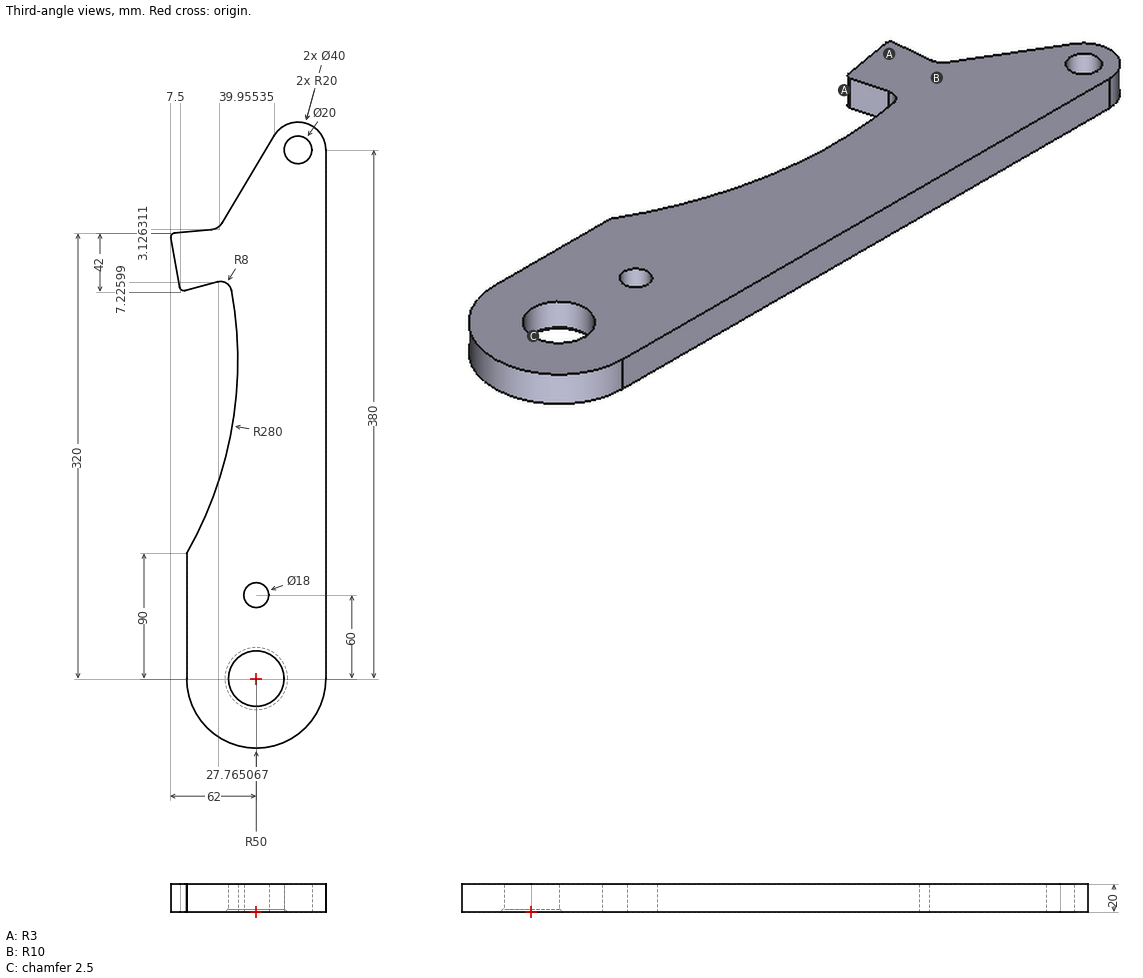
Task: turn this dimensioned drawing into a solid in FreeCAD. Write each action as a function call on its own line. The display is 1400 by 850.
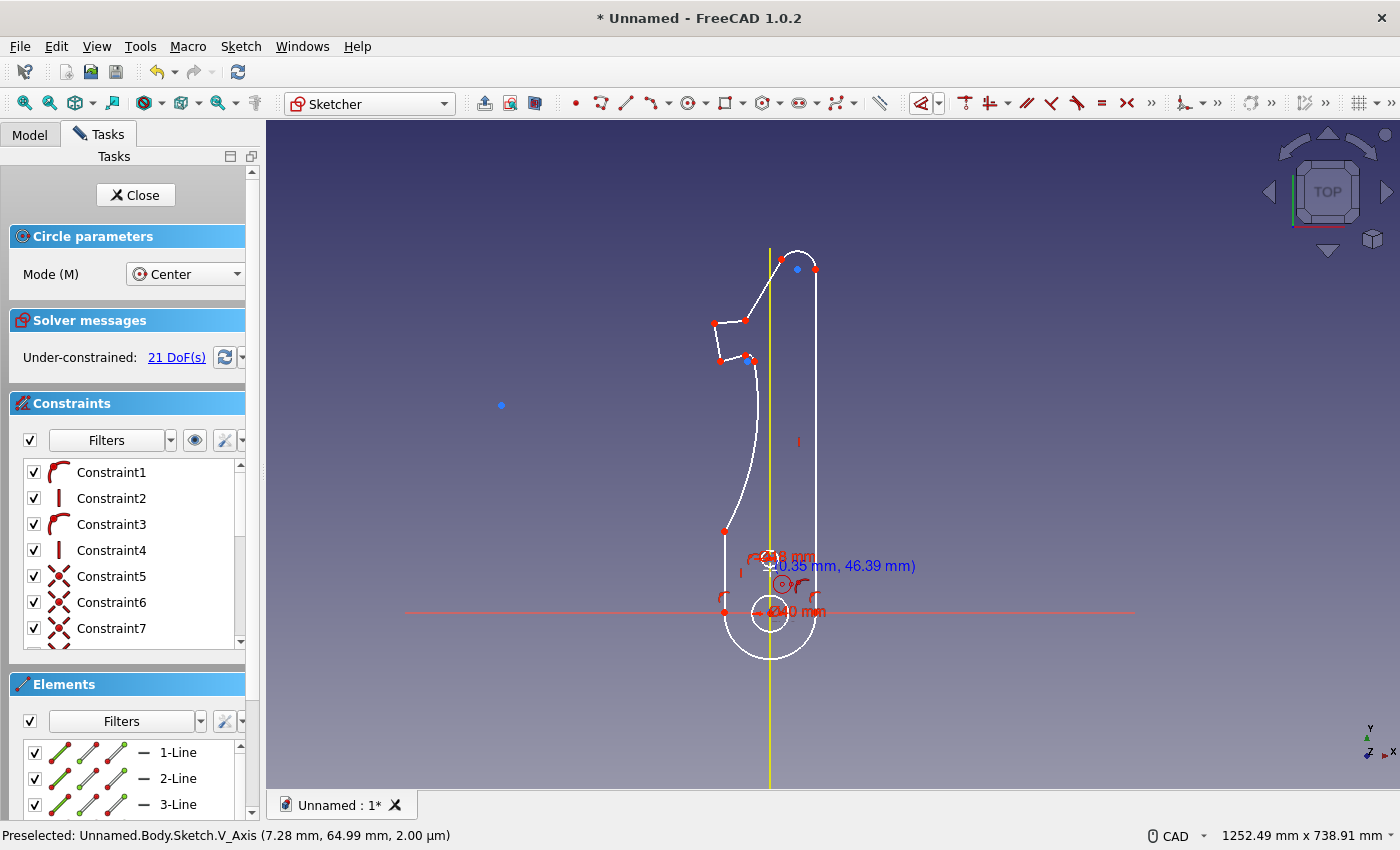
scroll(797, 269, up, 5)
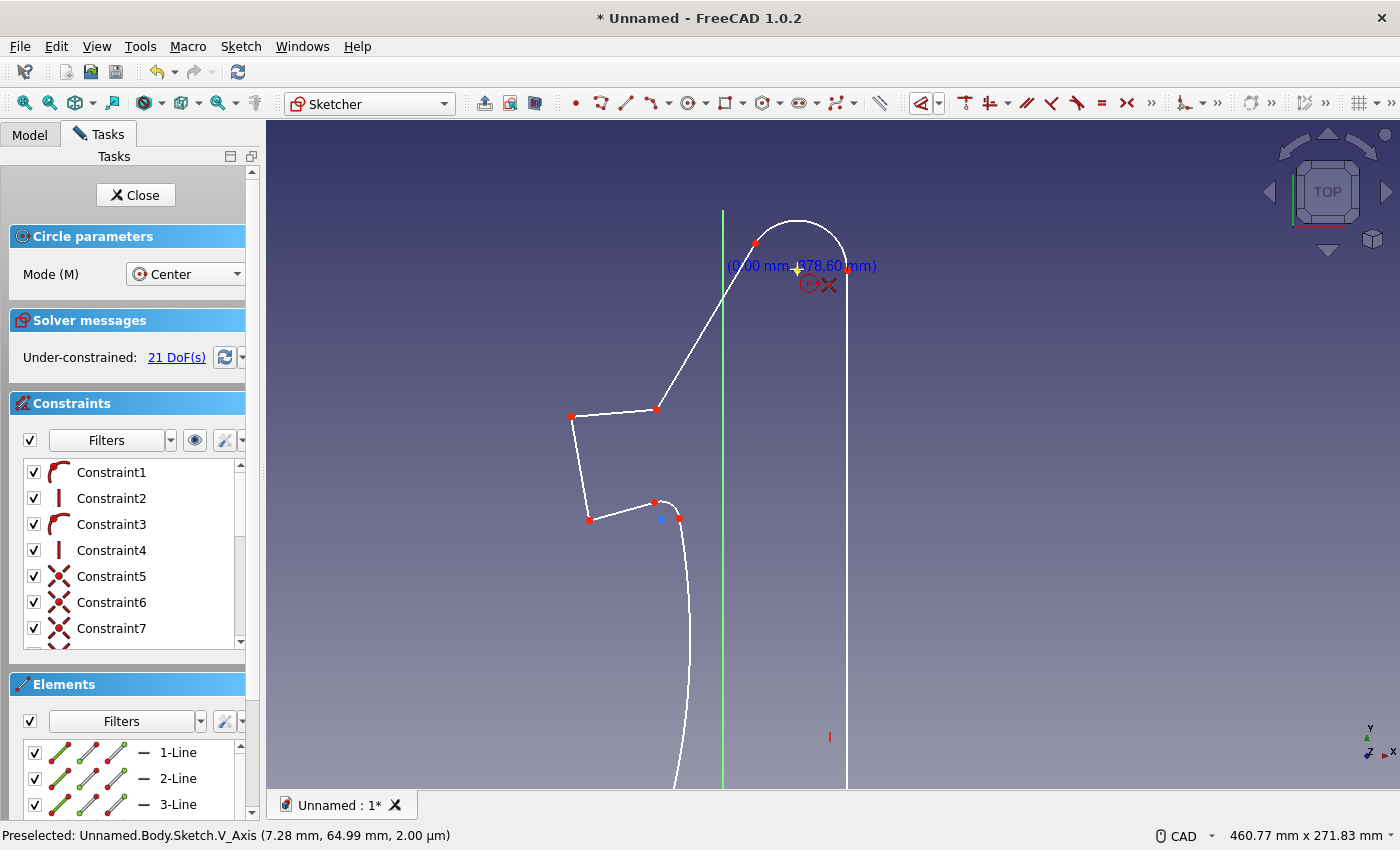
click(797, 268)
move(814, 250)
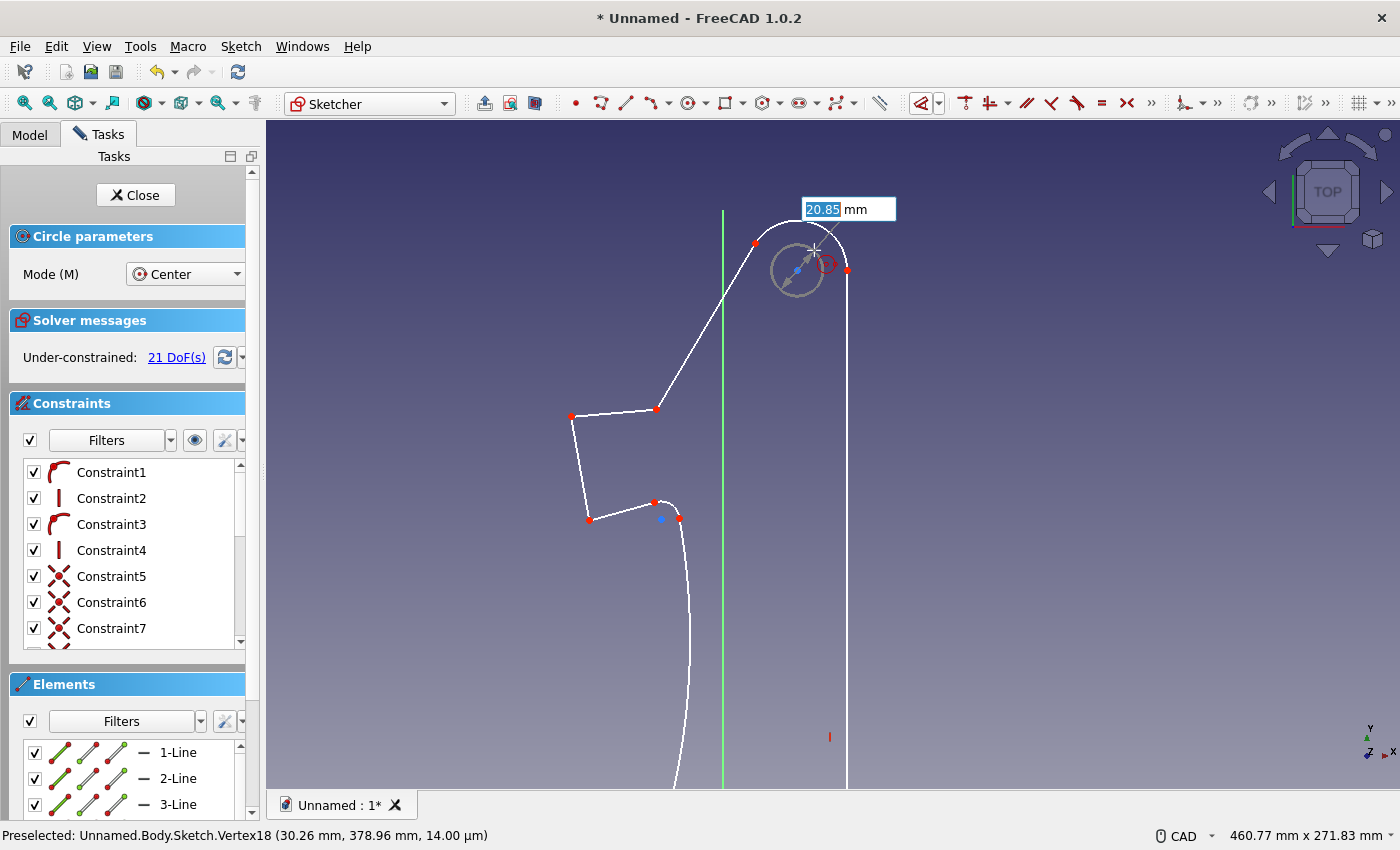
text(20)
key(Return)
key(Escape)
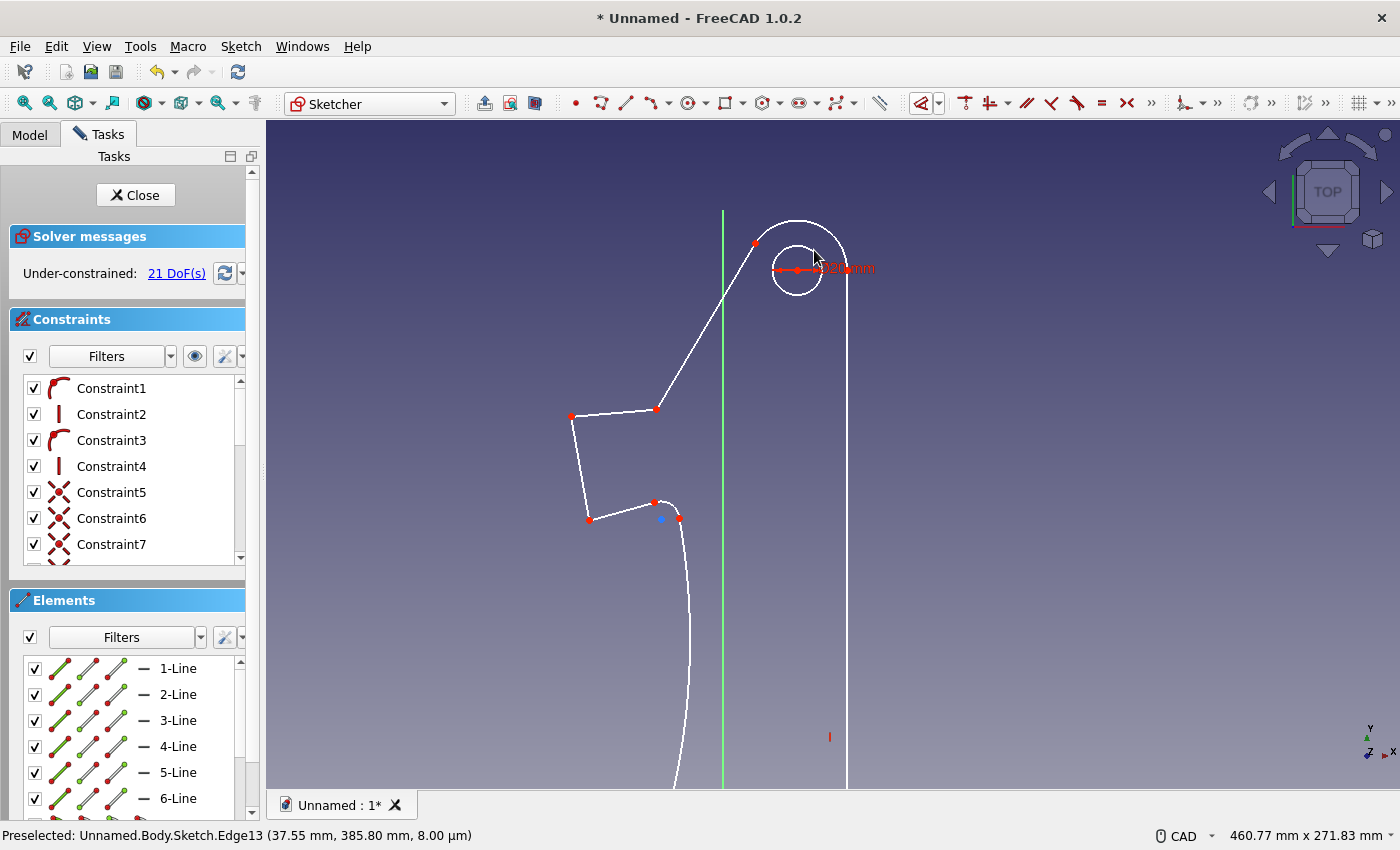
click(847, 550)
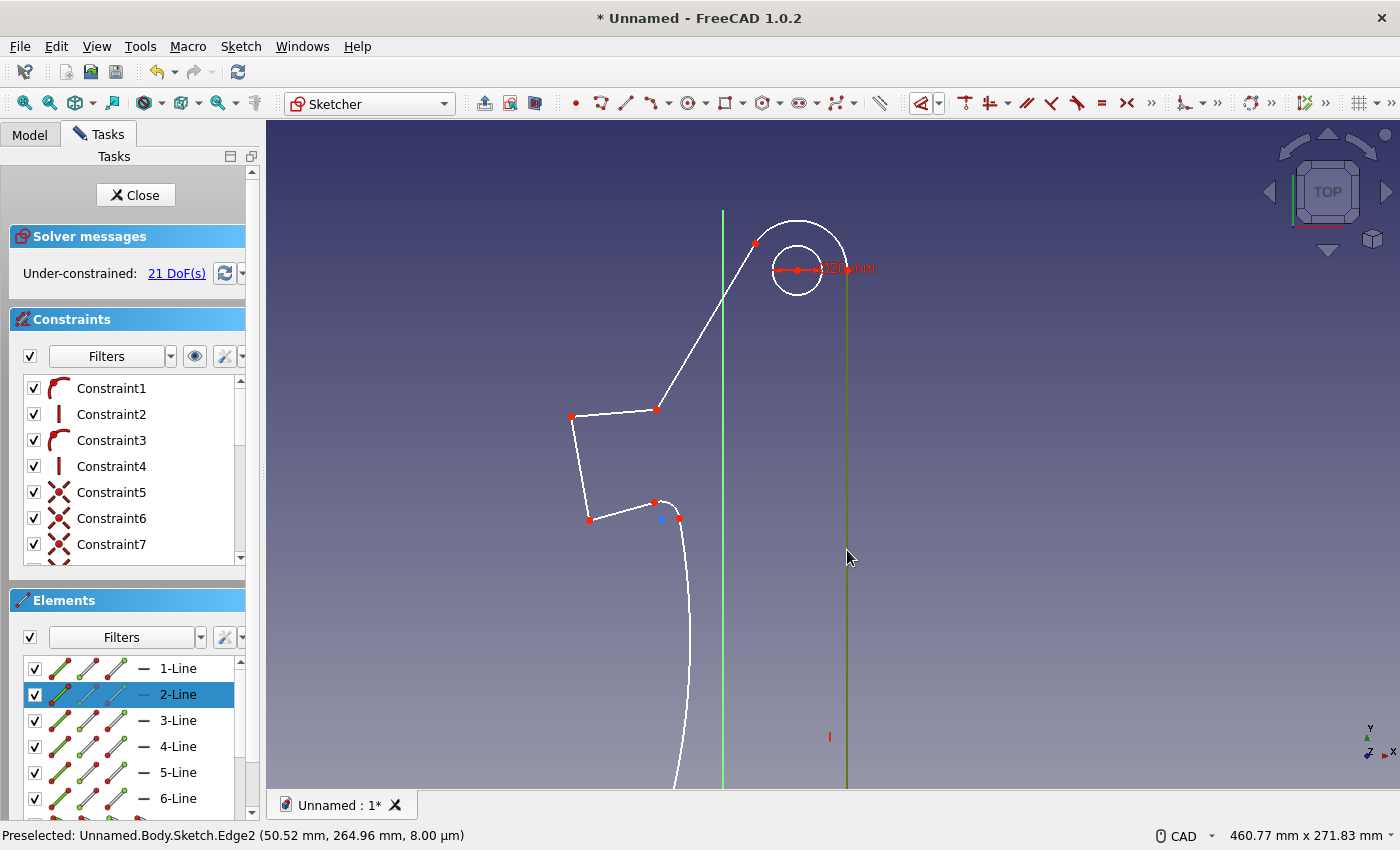
click(833, 236)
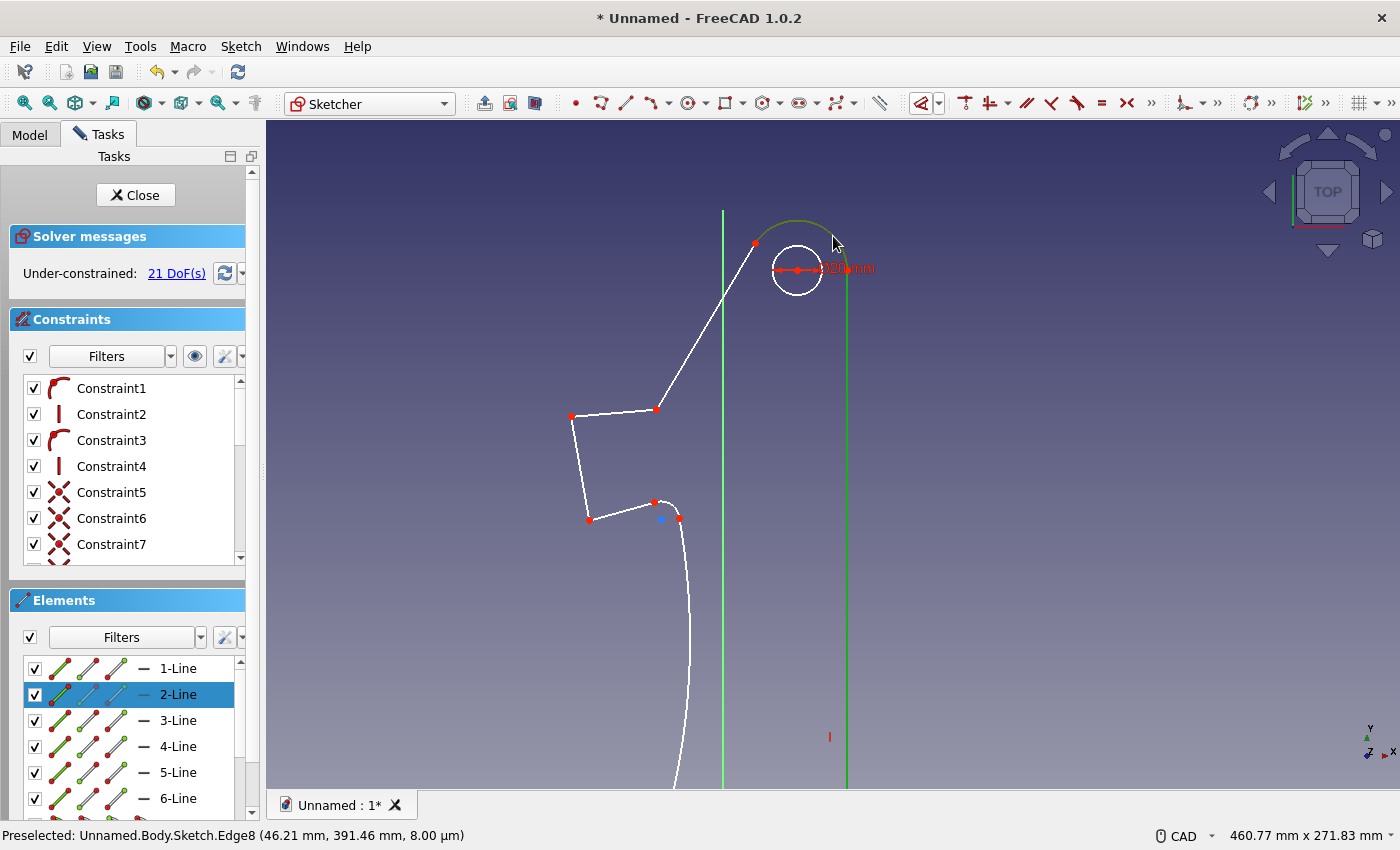
click(1077, 104)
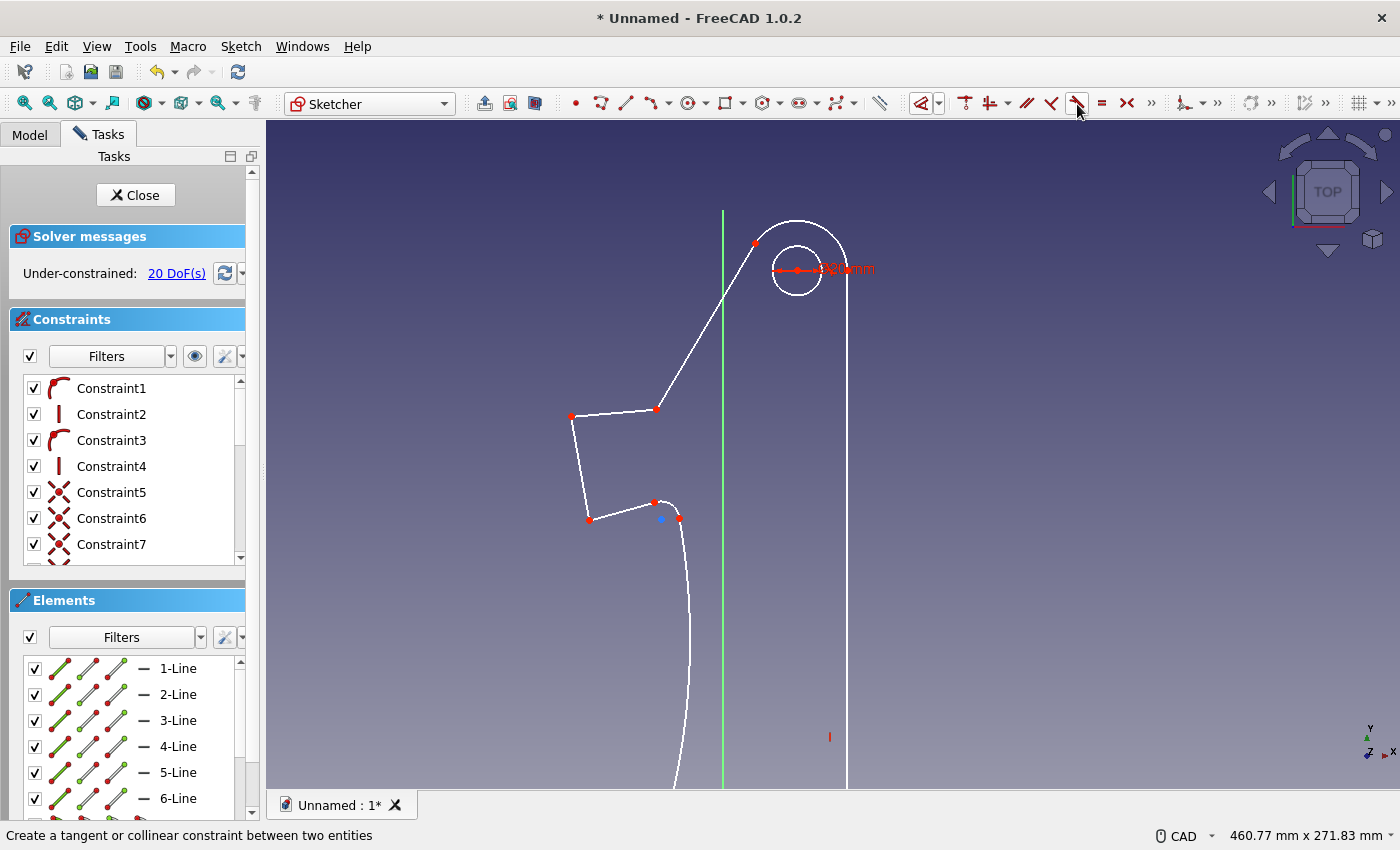
click(726, 294)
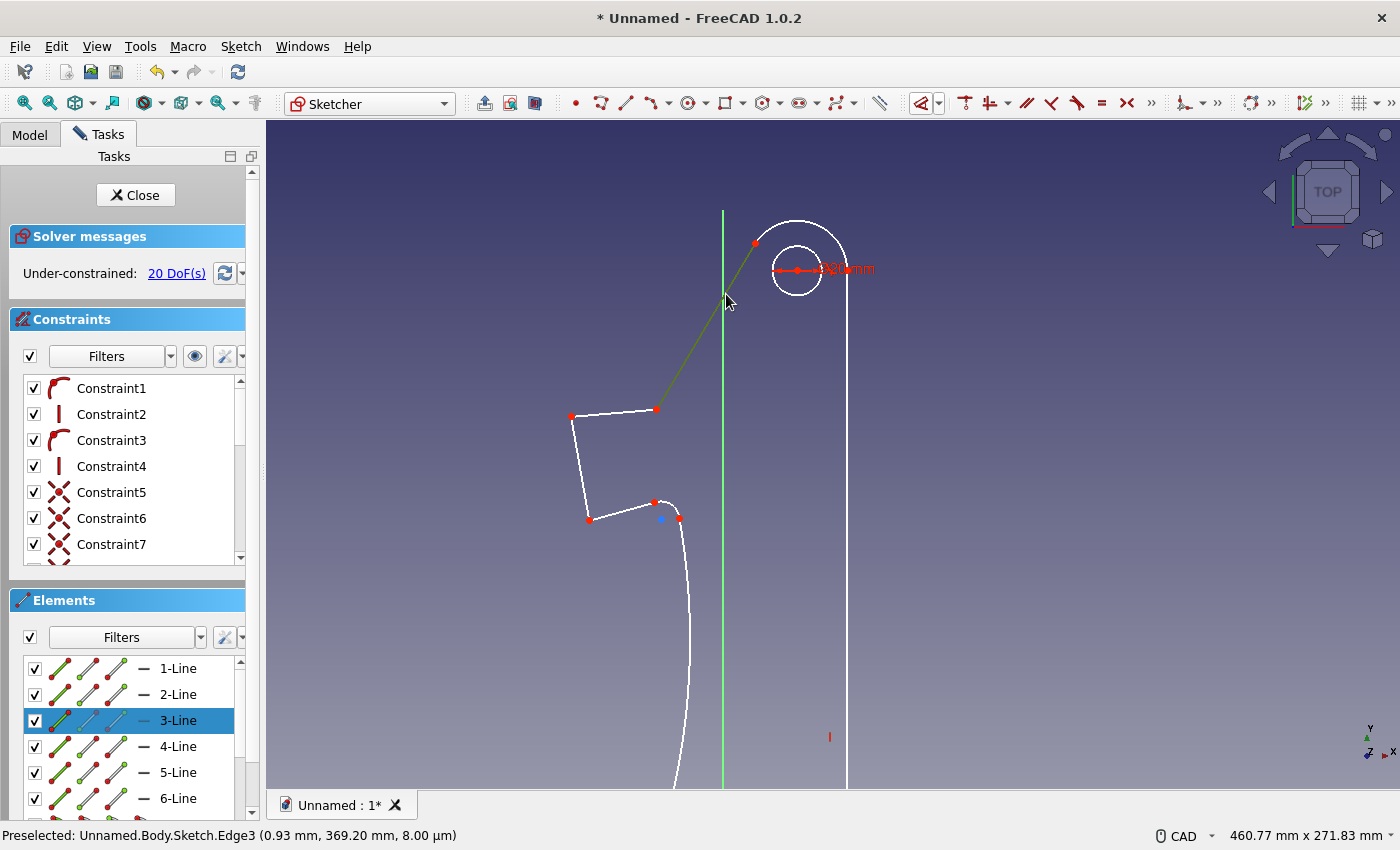
click(833, 236)